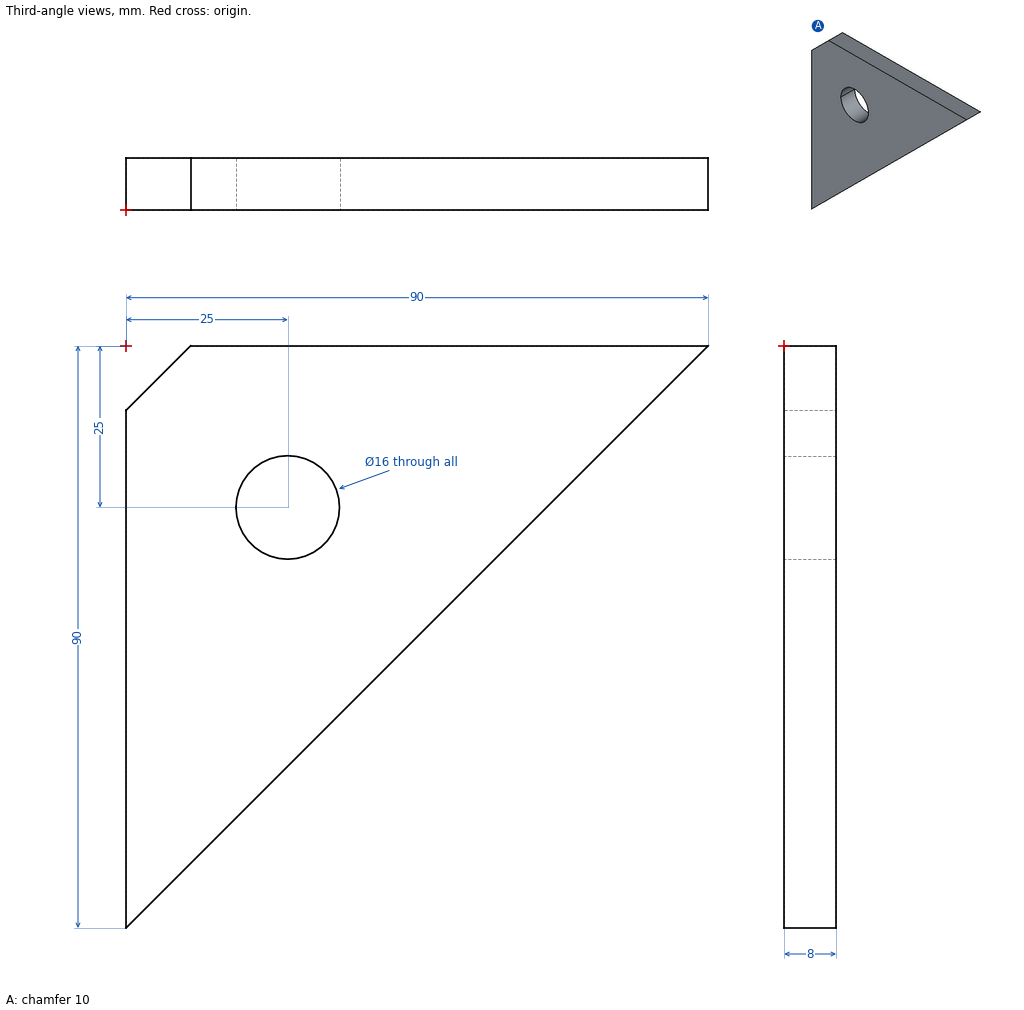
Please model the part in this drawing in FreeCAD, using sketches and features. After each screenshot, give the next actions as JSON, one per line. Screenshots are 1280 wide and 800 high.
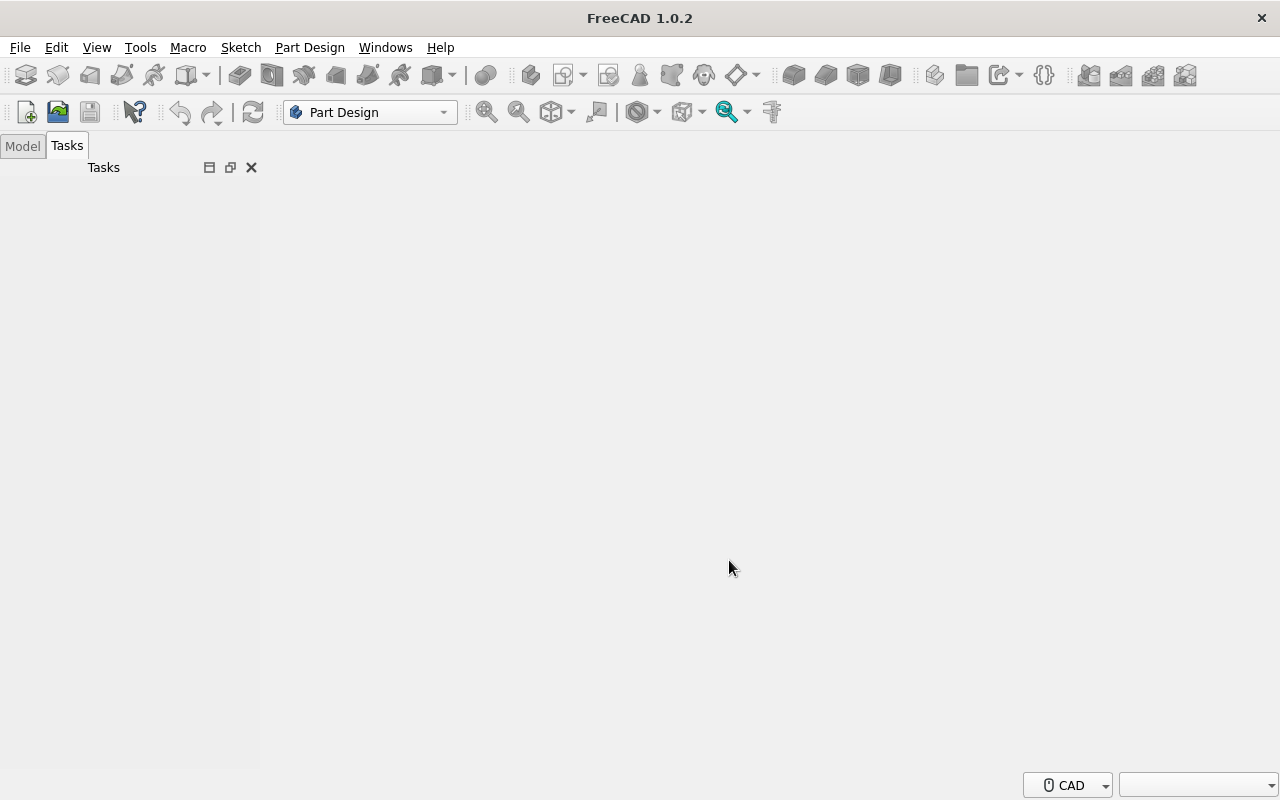
{"action": "key", "text": "ctrl+n"}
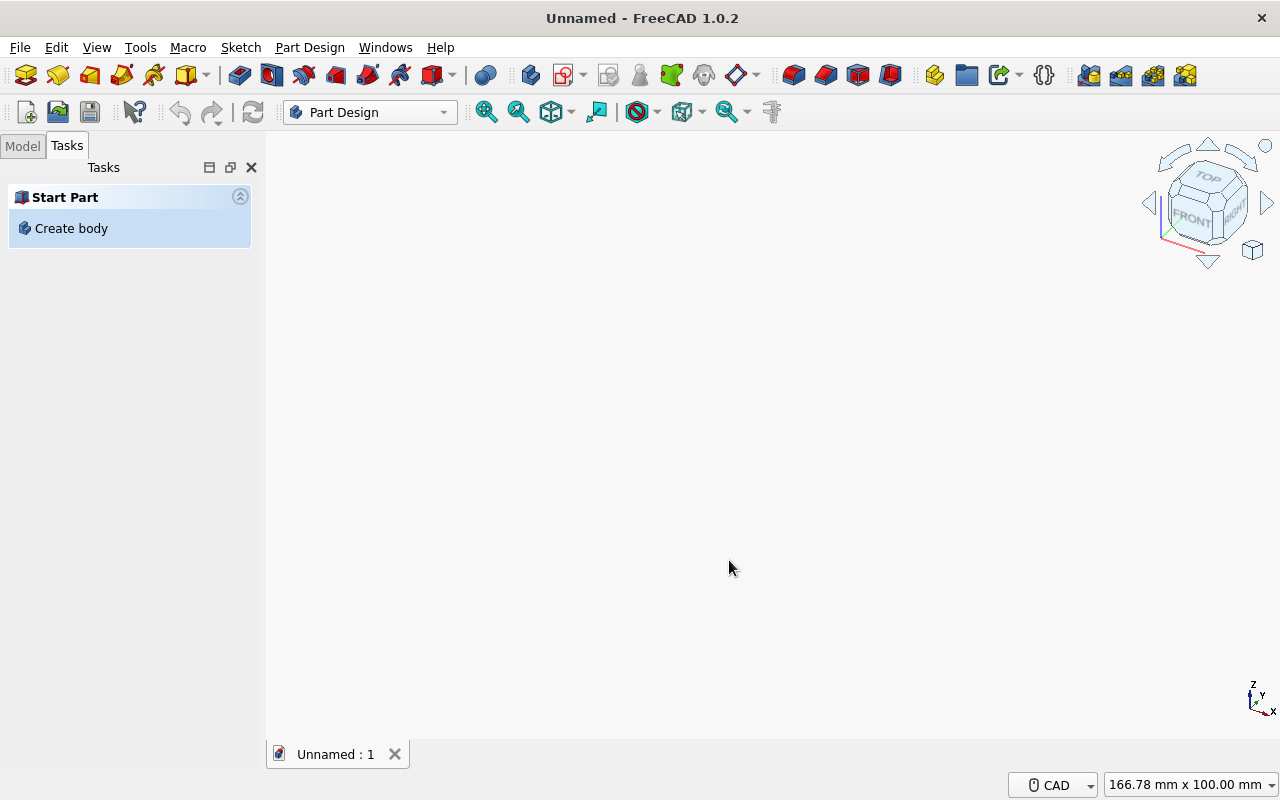
{"action": "left_click", "coordinate": [564, 76]}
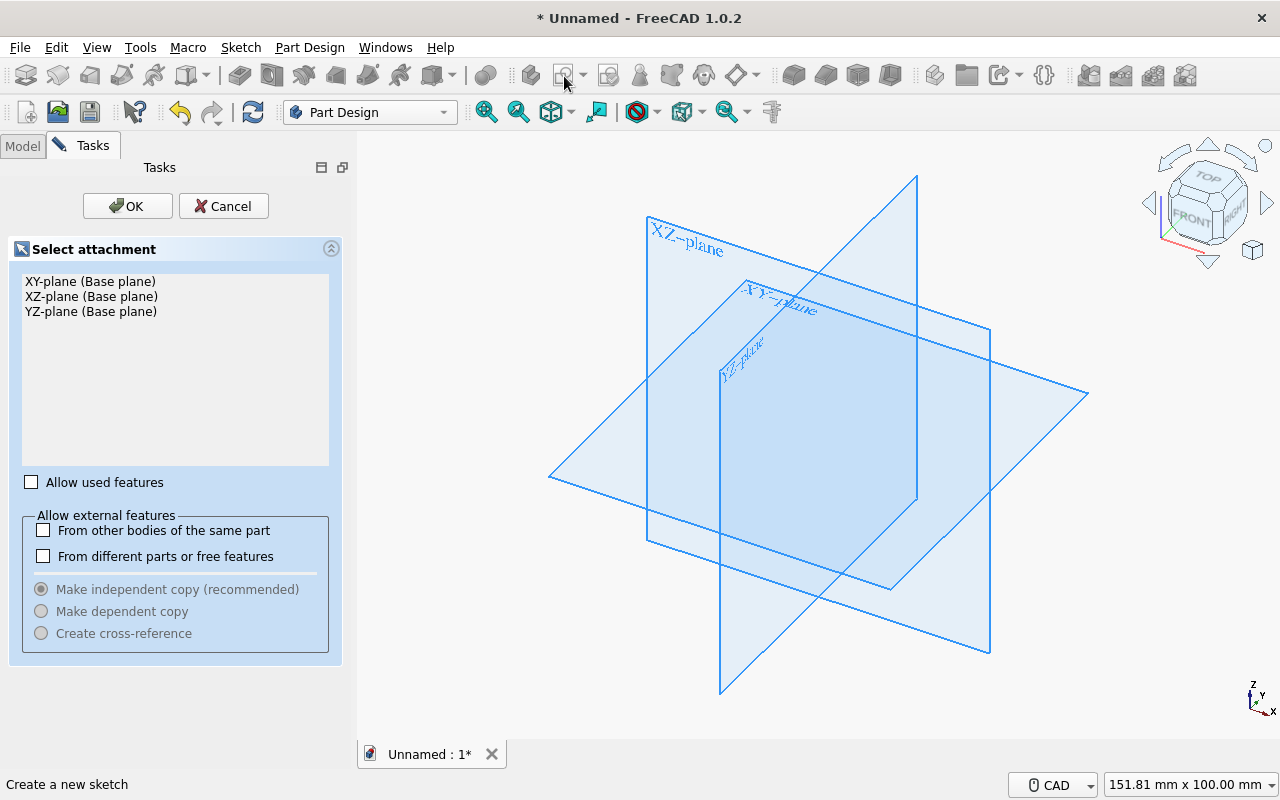
{"action": "left_click", "coordinate": [82, 296]}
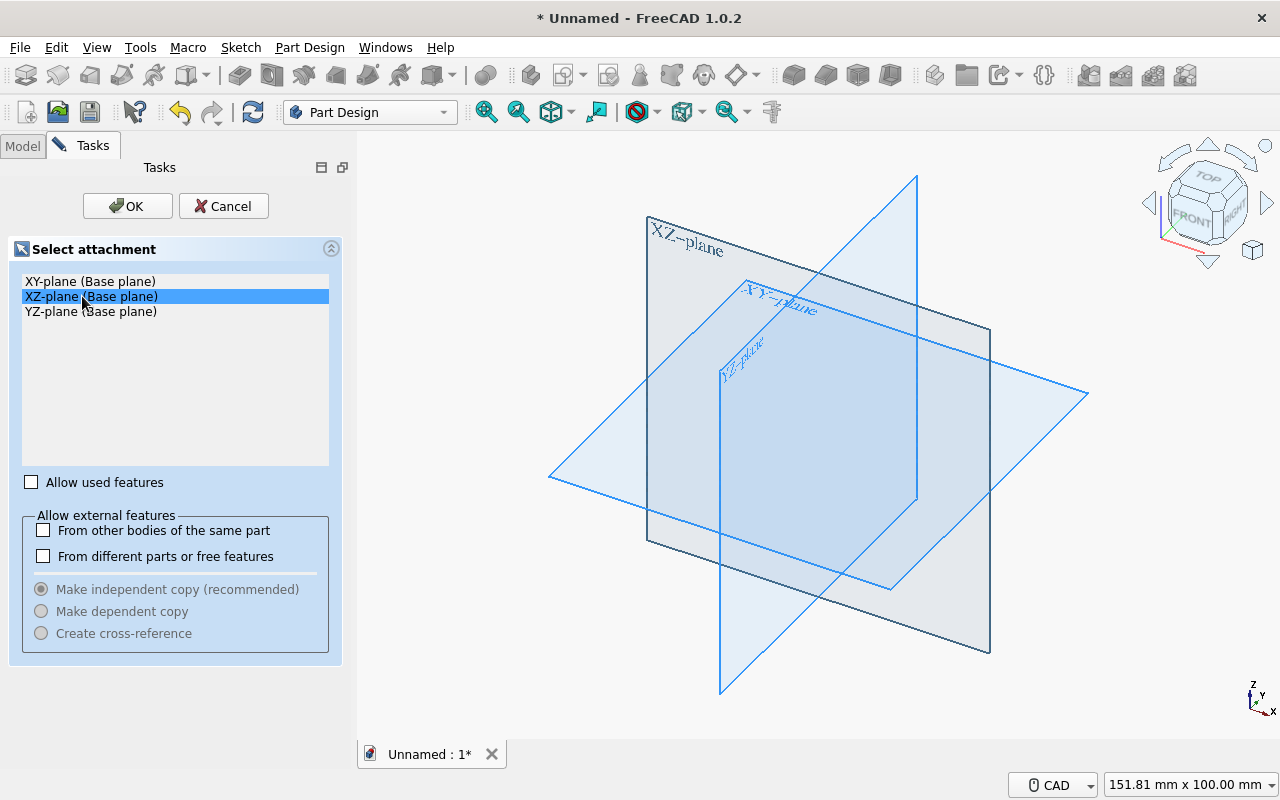
{"action": "left_click", "coordinate": [128, 206]}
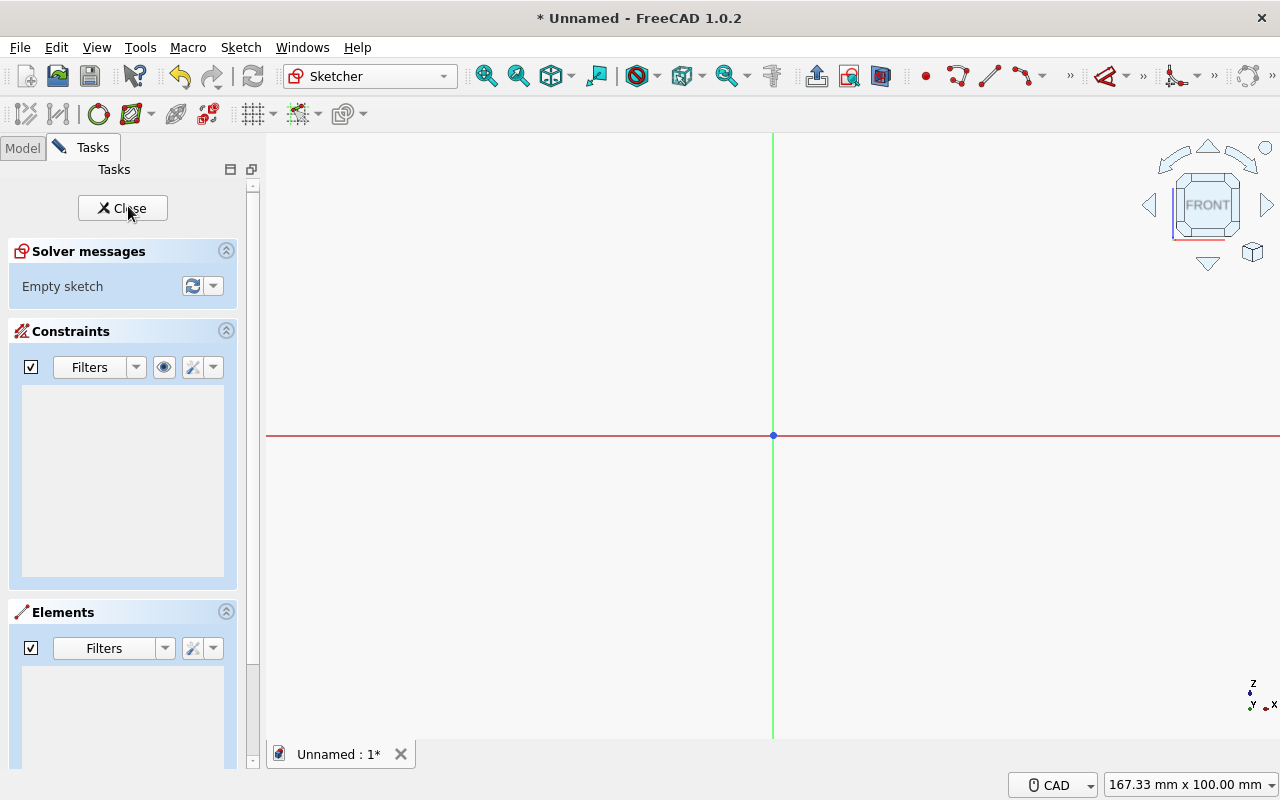
{"action": "scroll", "coordinate": [294, 161], "scroll_direction": "down", "scroll_amount": 3}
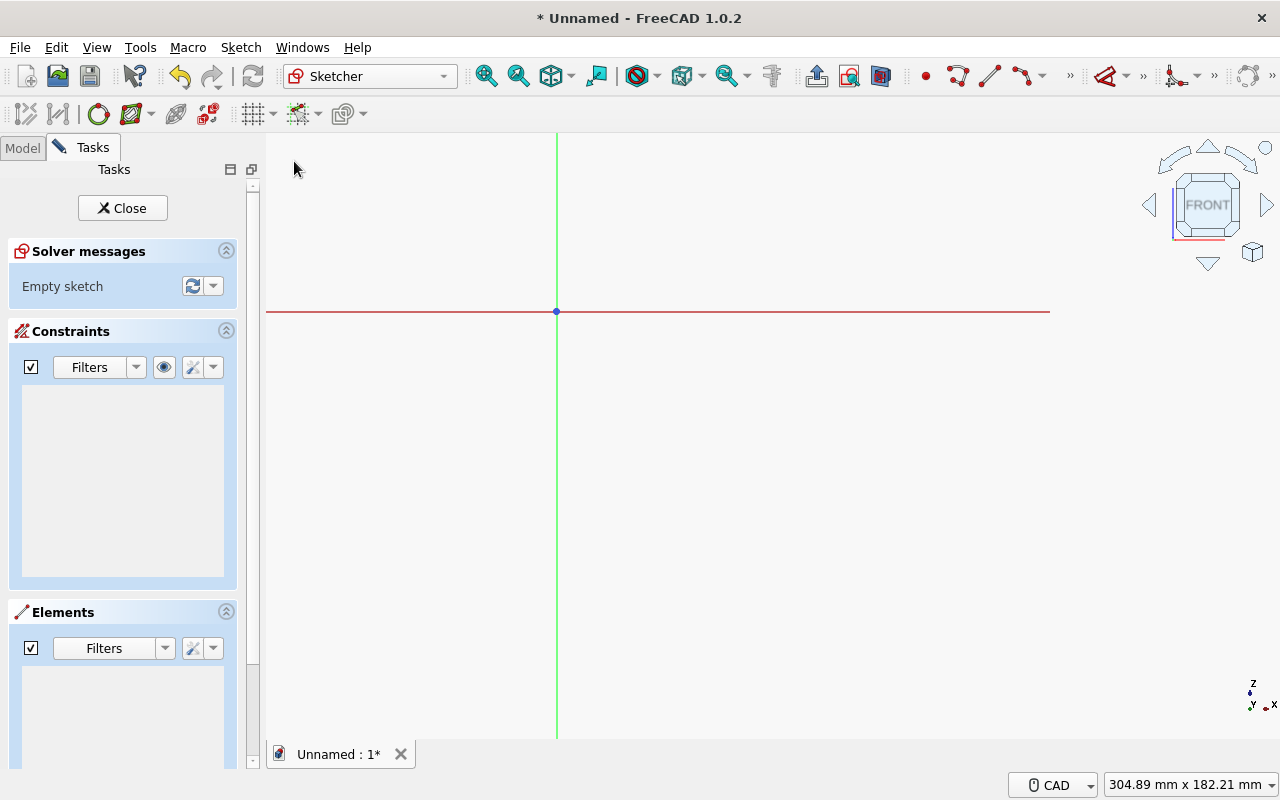
{"action": "left_click", "coordinate": [958, 76]}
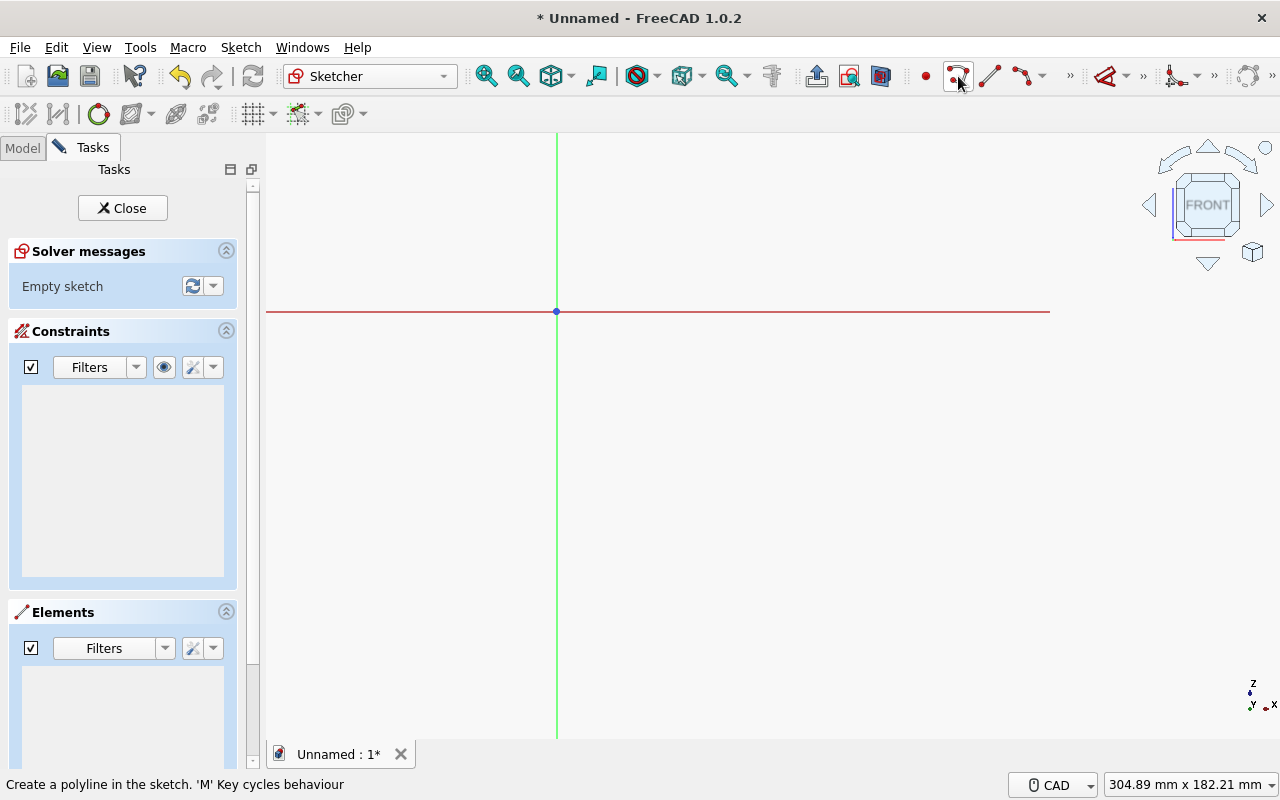
{"action": "left_click", "coordinate": [557, 312]}
{"action": "left_click", "coordinate": [856, 321]}
{"action": "left_click", "coordinate": [566, 611]}
{"action": "left_click", "coordinate": [557, 312]}
{"action": "key", "text": "Escape"}
{"action": "key", "text": "Escape"}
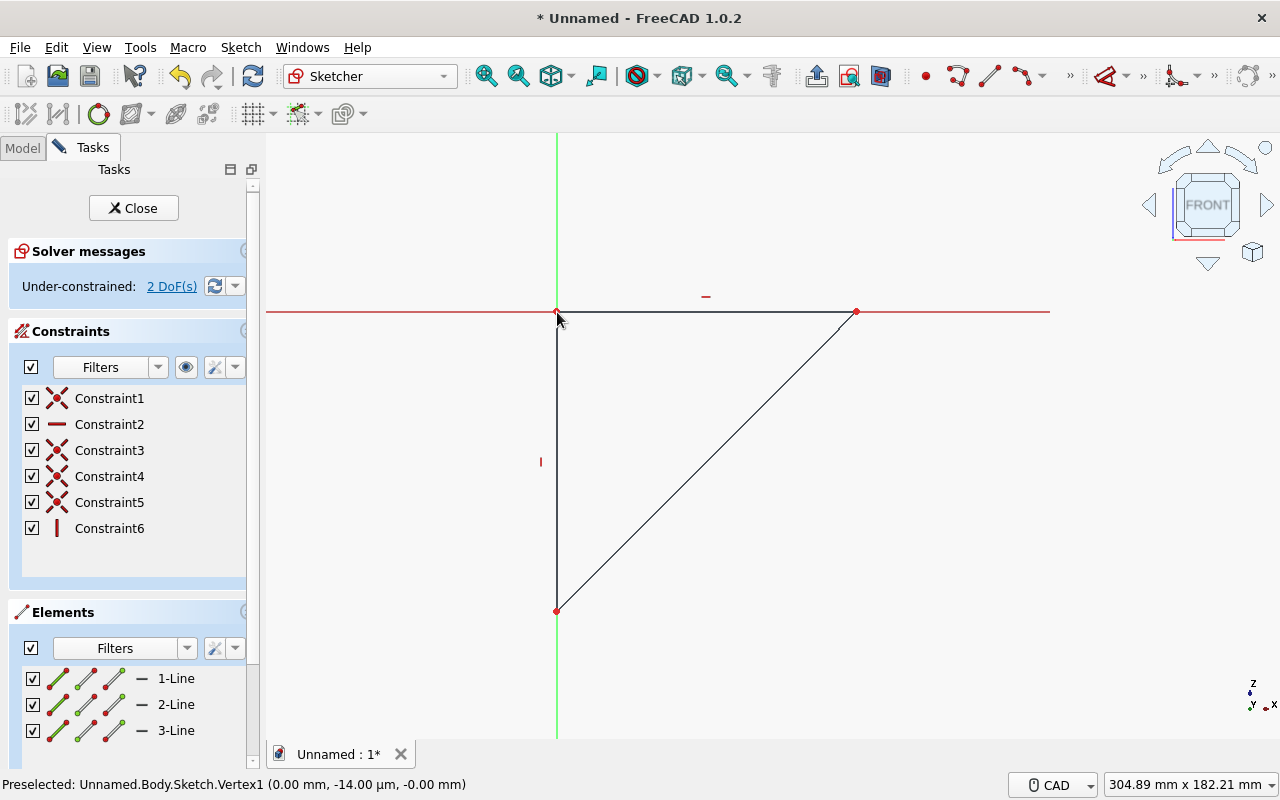
{"action": "left_click", "coordinate": [1106, 76]}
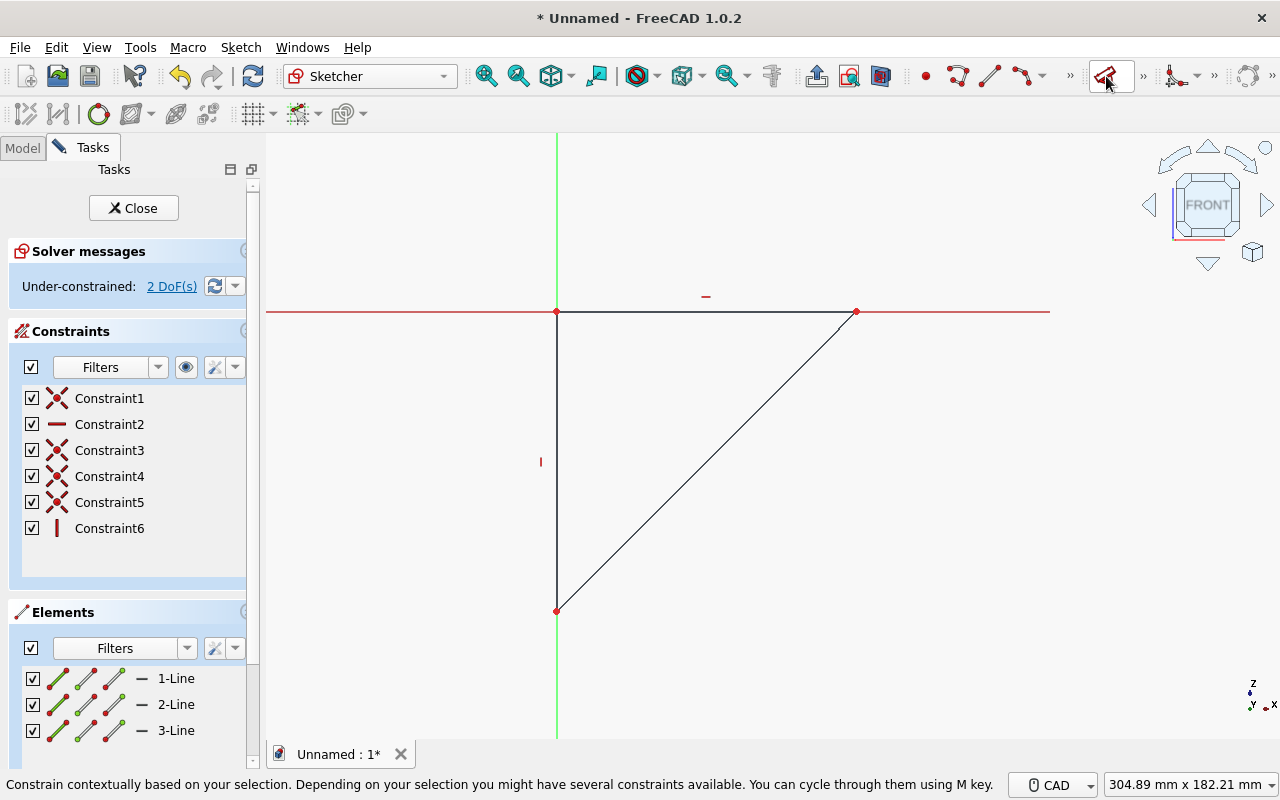
{"action": "left_click", "coordinate": [647, 312]}
{"action": "left_click", "coordinate": [706, 278]}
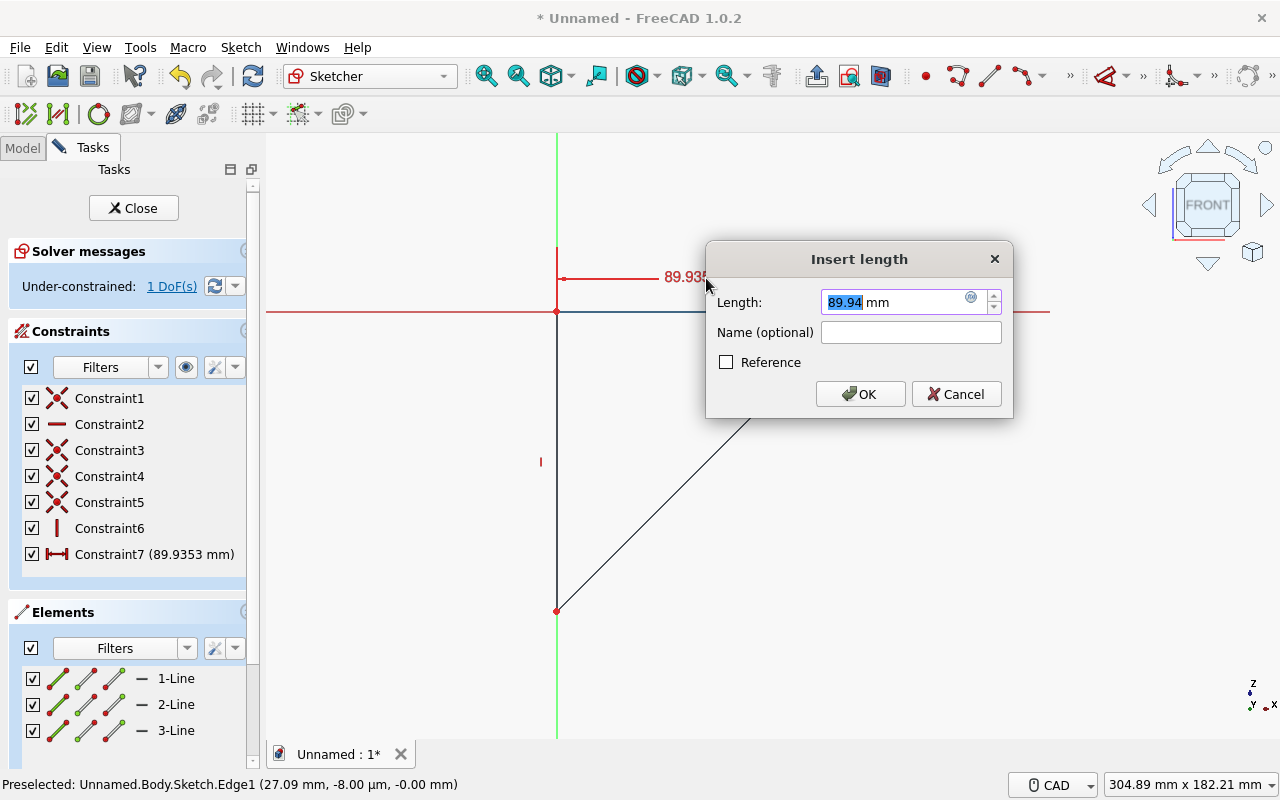
{"action": "type", "text": "90"}
{"action": "key", "text": "Return"}